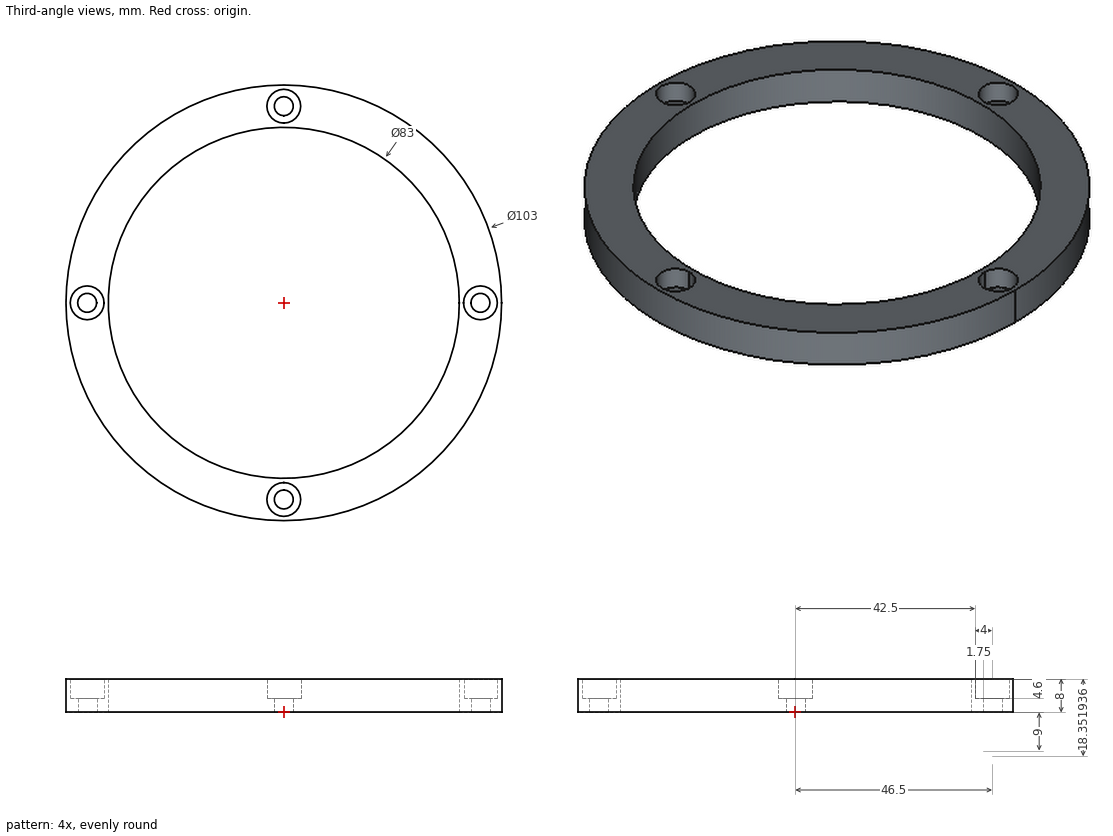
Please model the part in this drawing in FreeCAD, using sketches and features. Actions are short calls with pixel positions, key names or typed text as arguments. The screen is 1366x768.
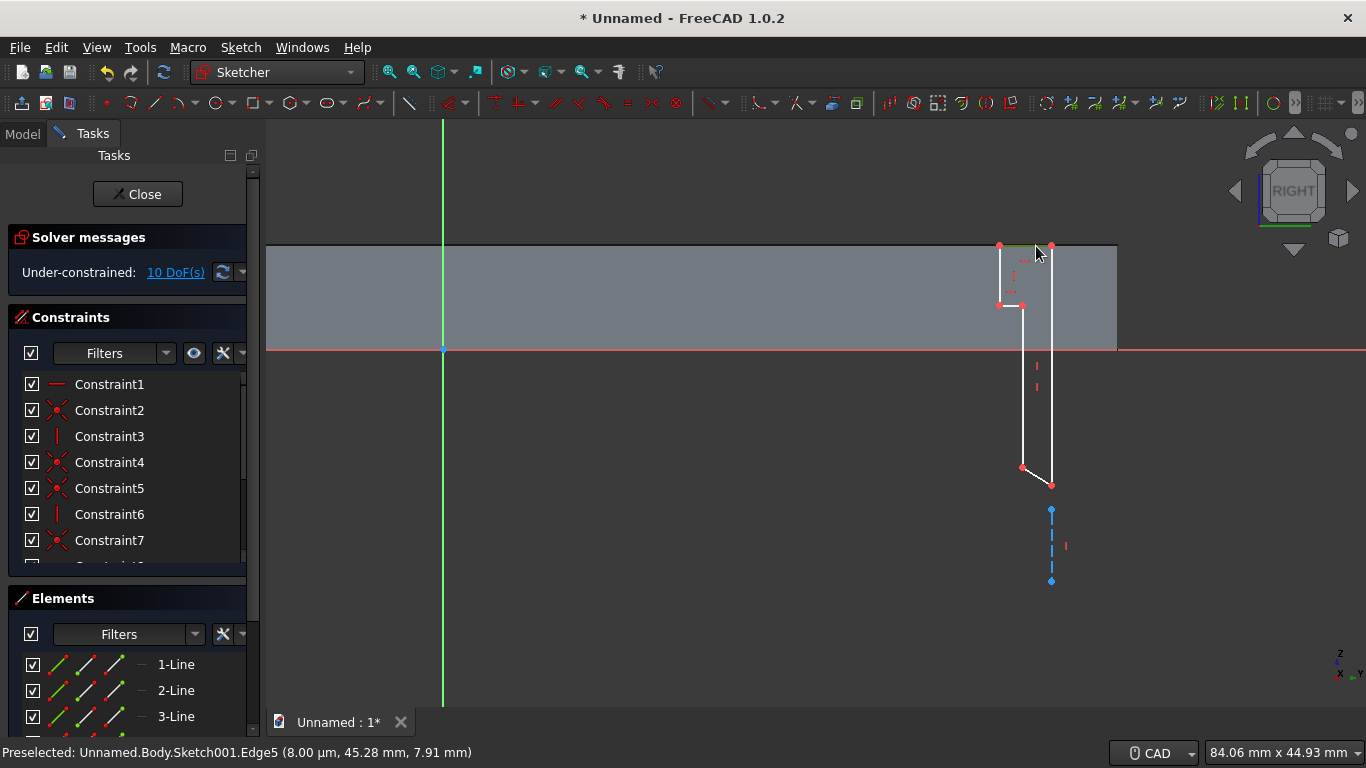
key(l)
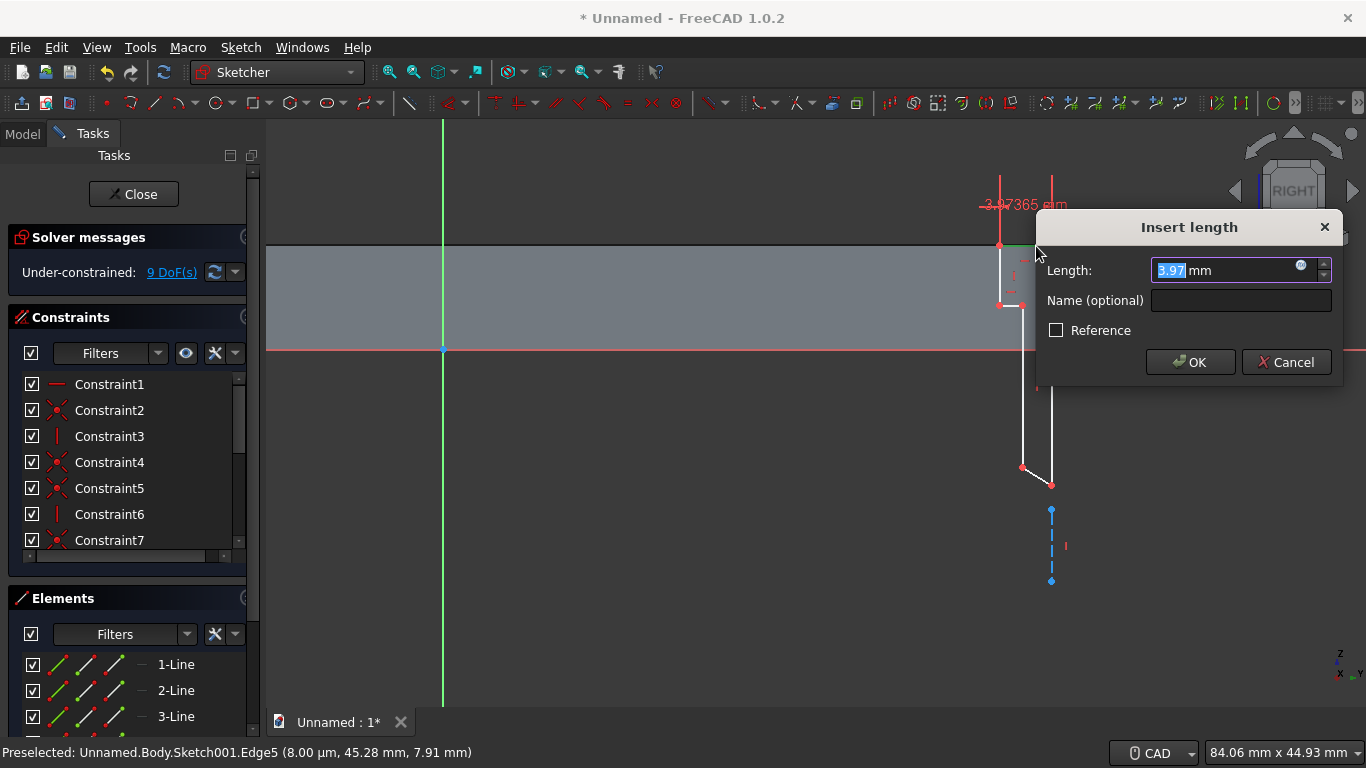
text(4)
key(Return)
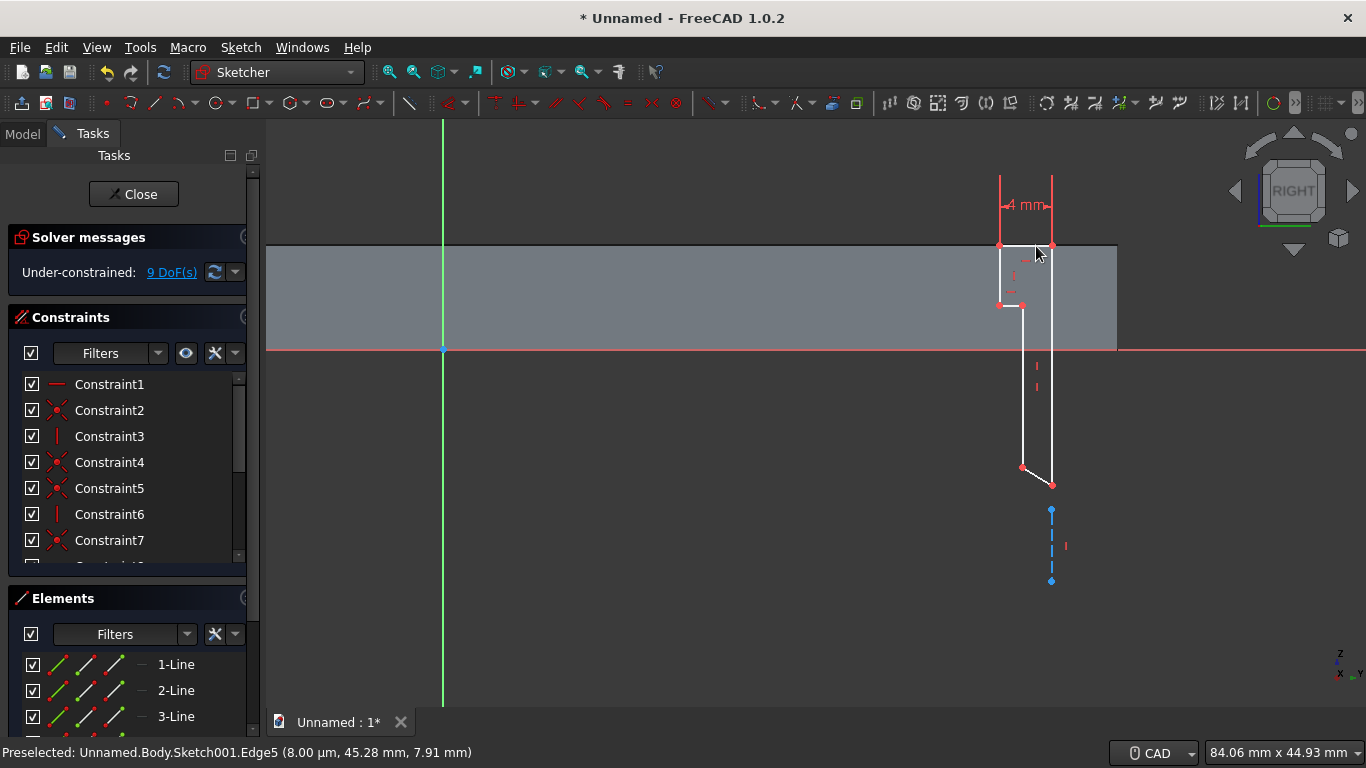
click(1023, 468)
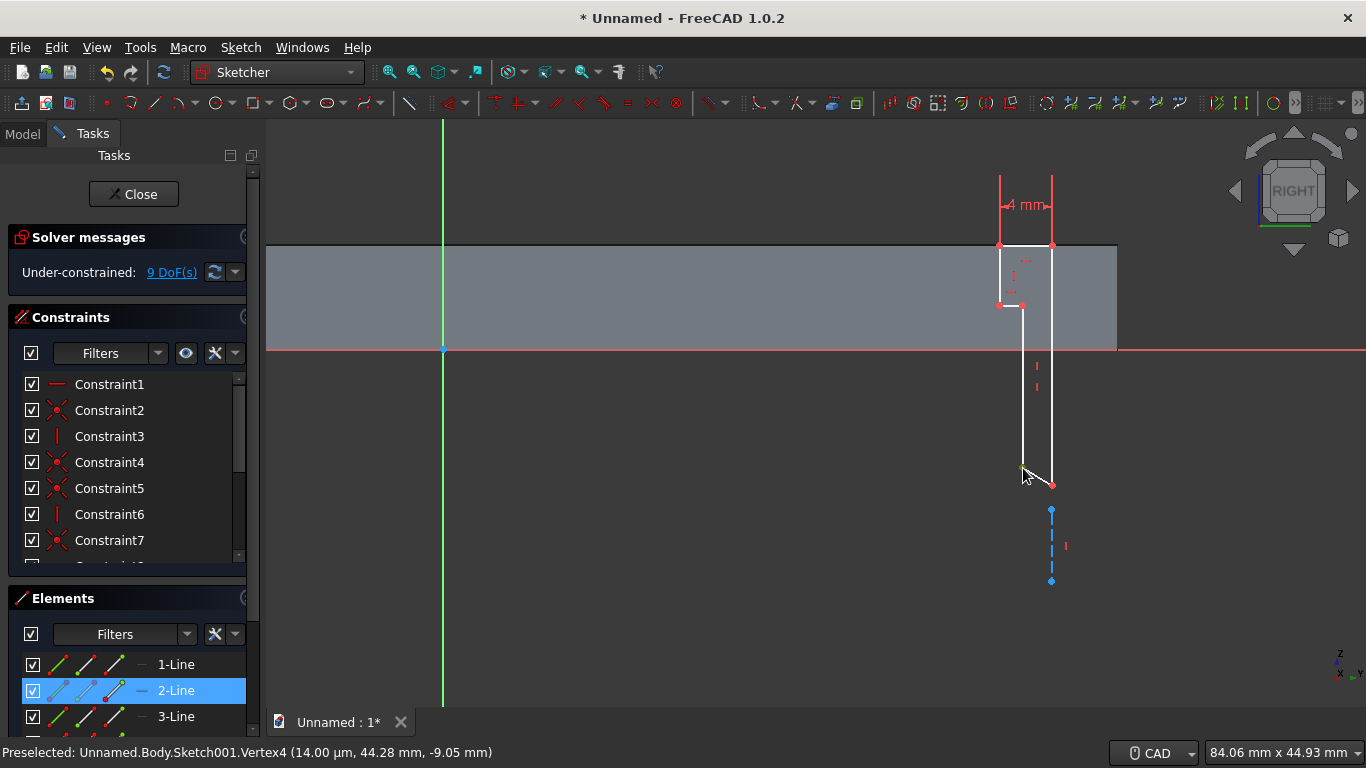
key(i)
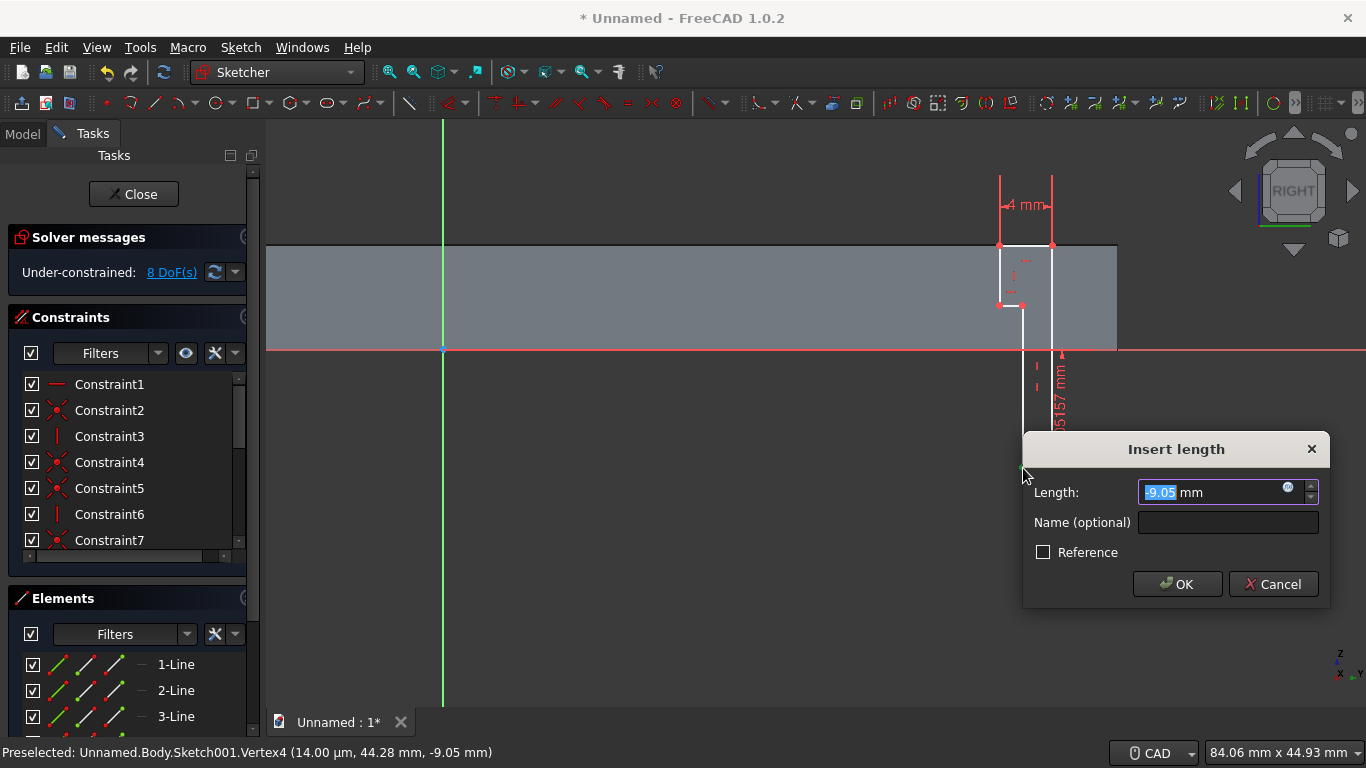
text(-9)
key(Return)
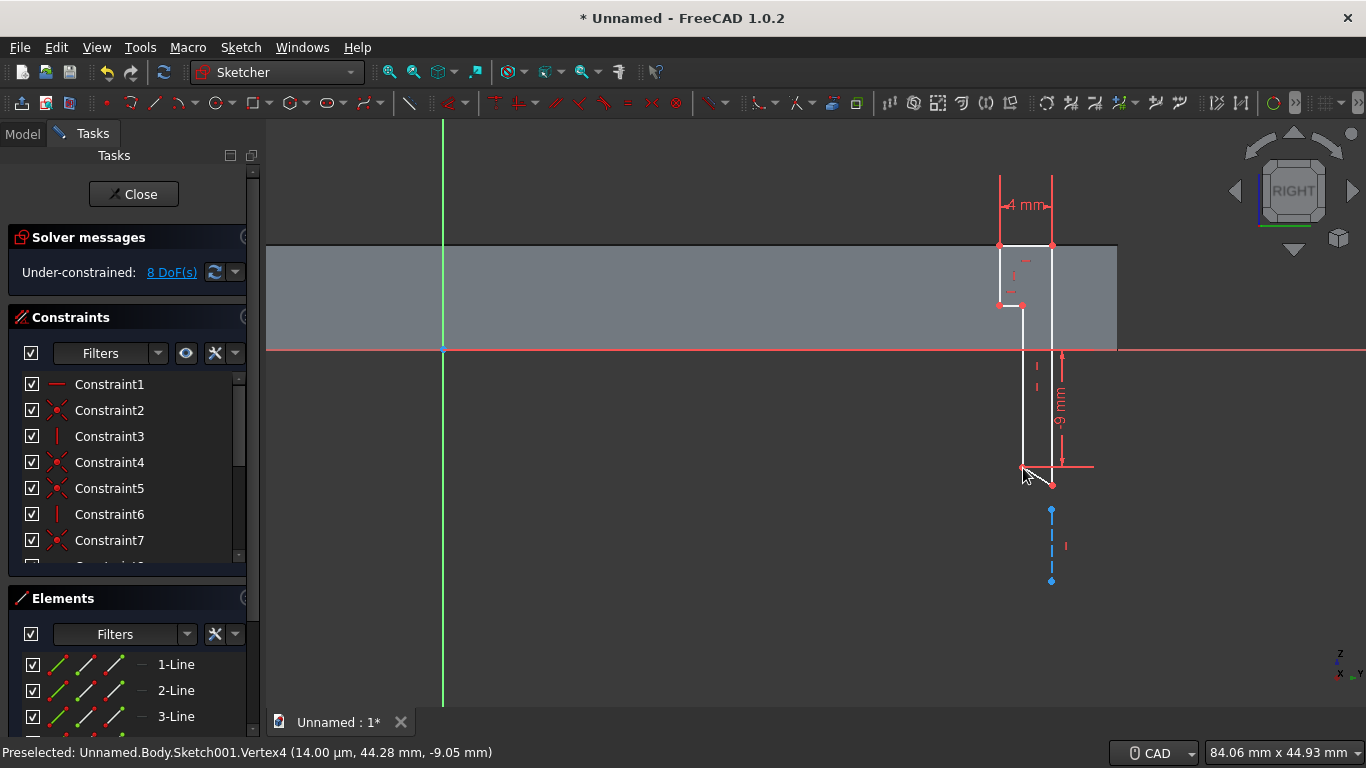
click(1052, 246)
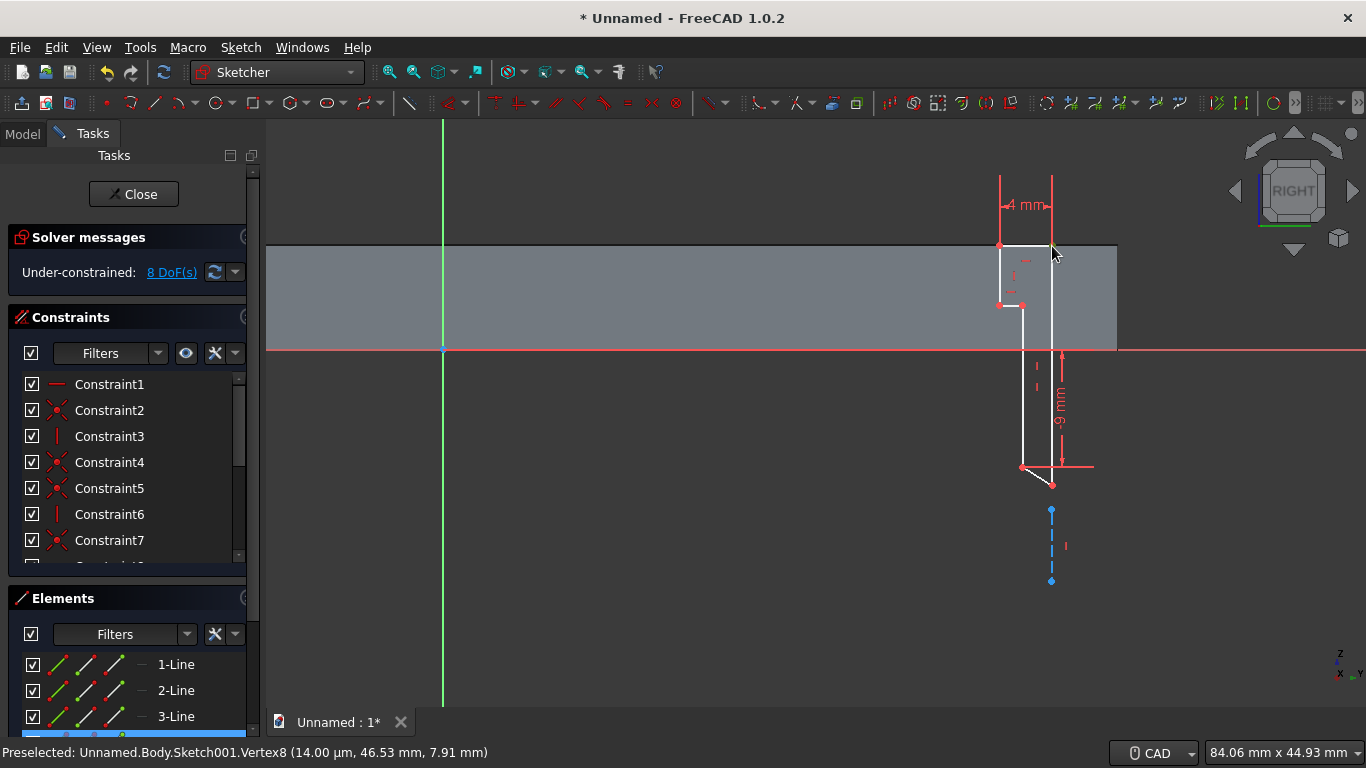
key(i)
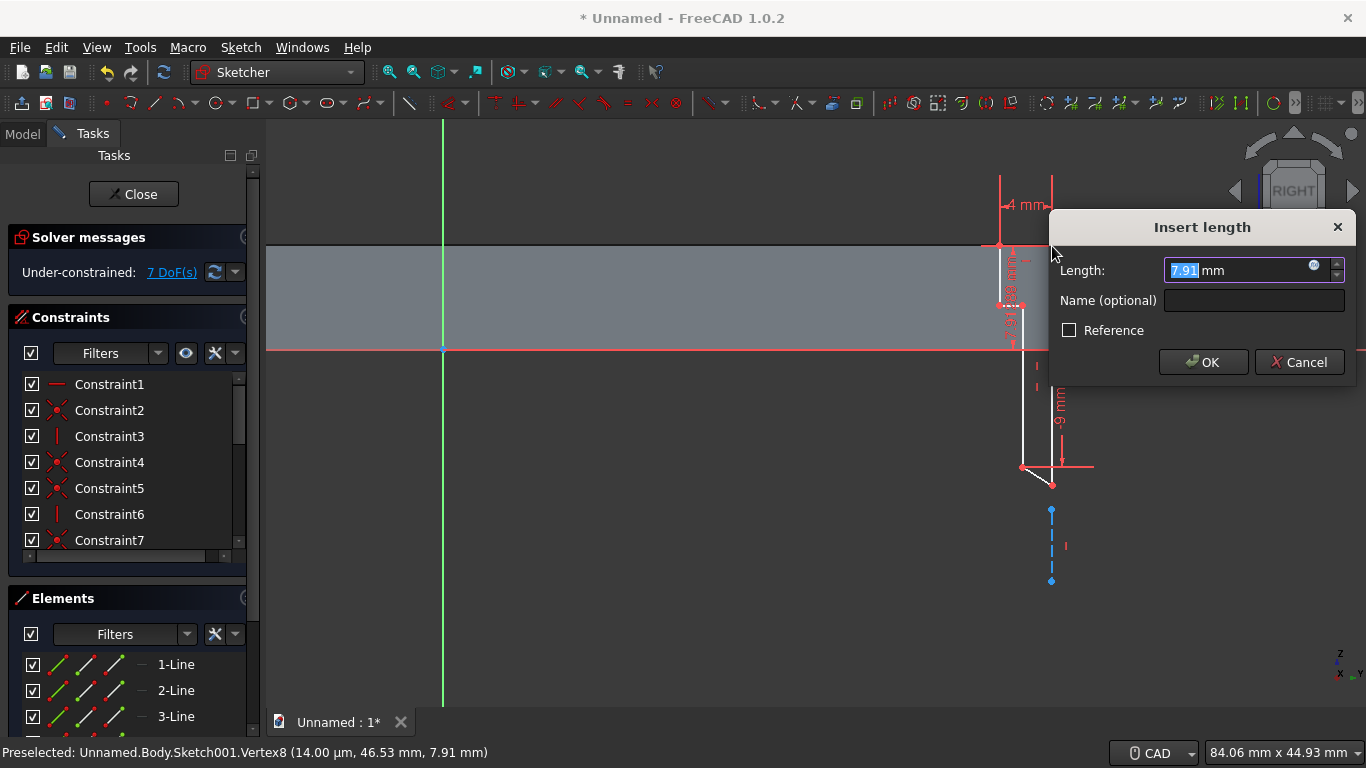
text(8)
key(Return)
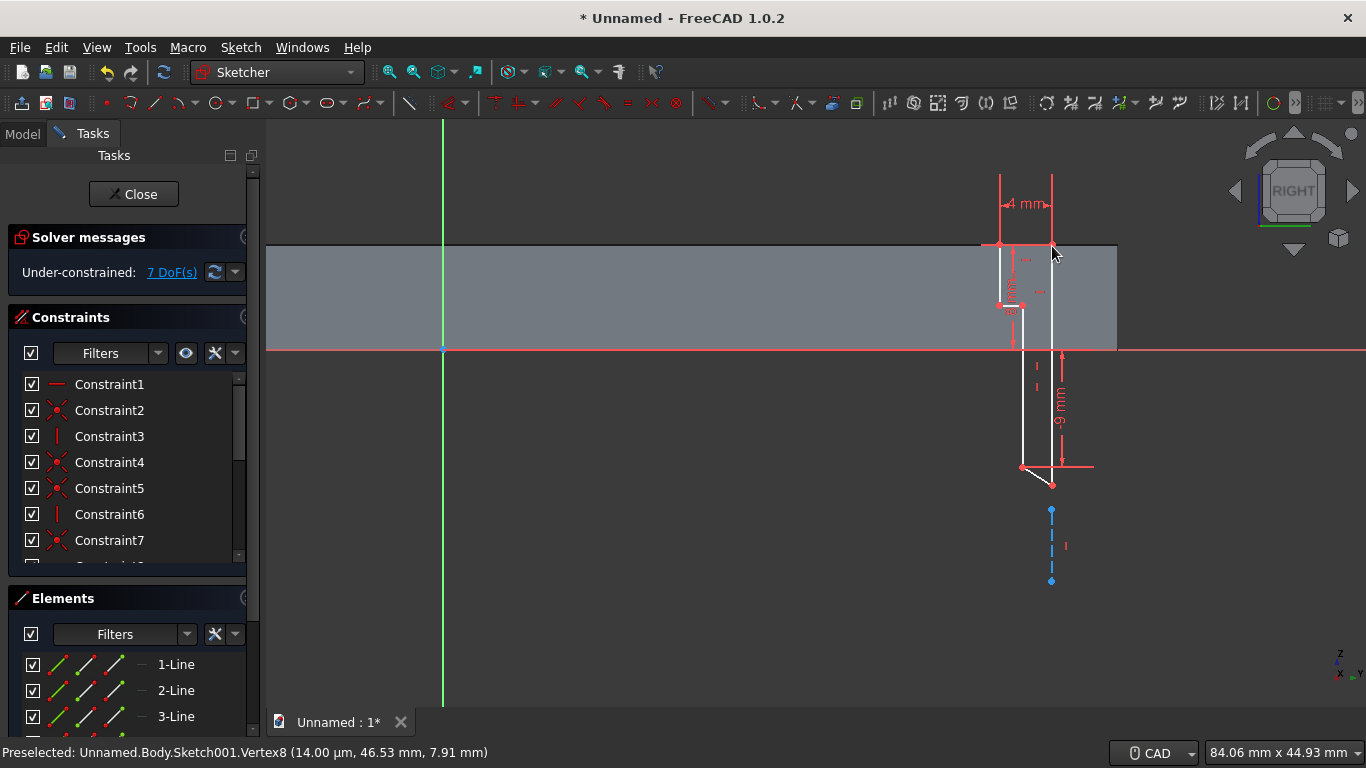
click(1000, 263)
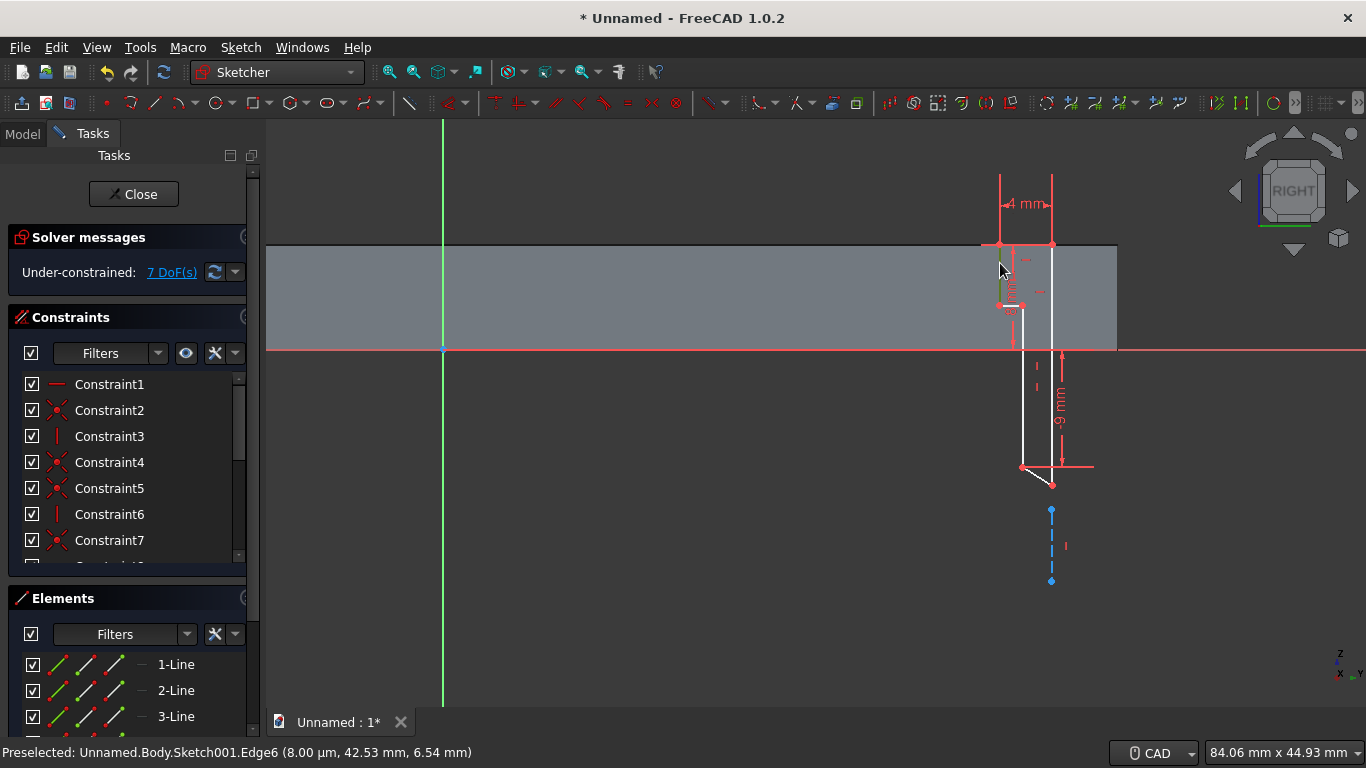
key(i)